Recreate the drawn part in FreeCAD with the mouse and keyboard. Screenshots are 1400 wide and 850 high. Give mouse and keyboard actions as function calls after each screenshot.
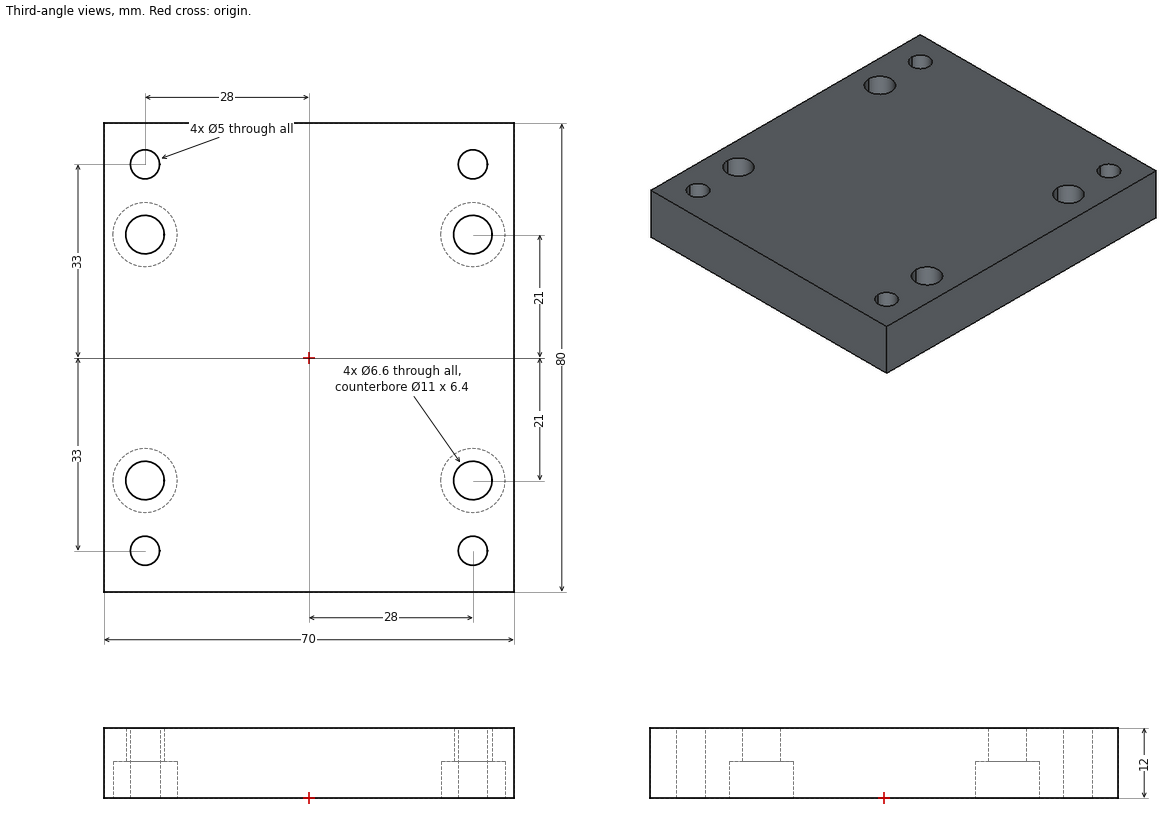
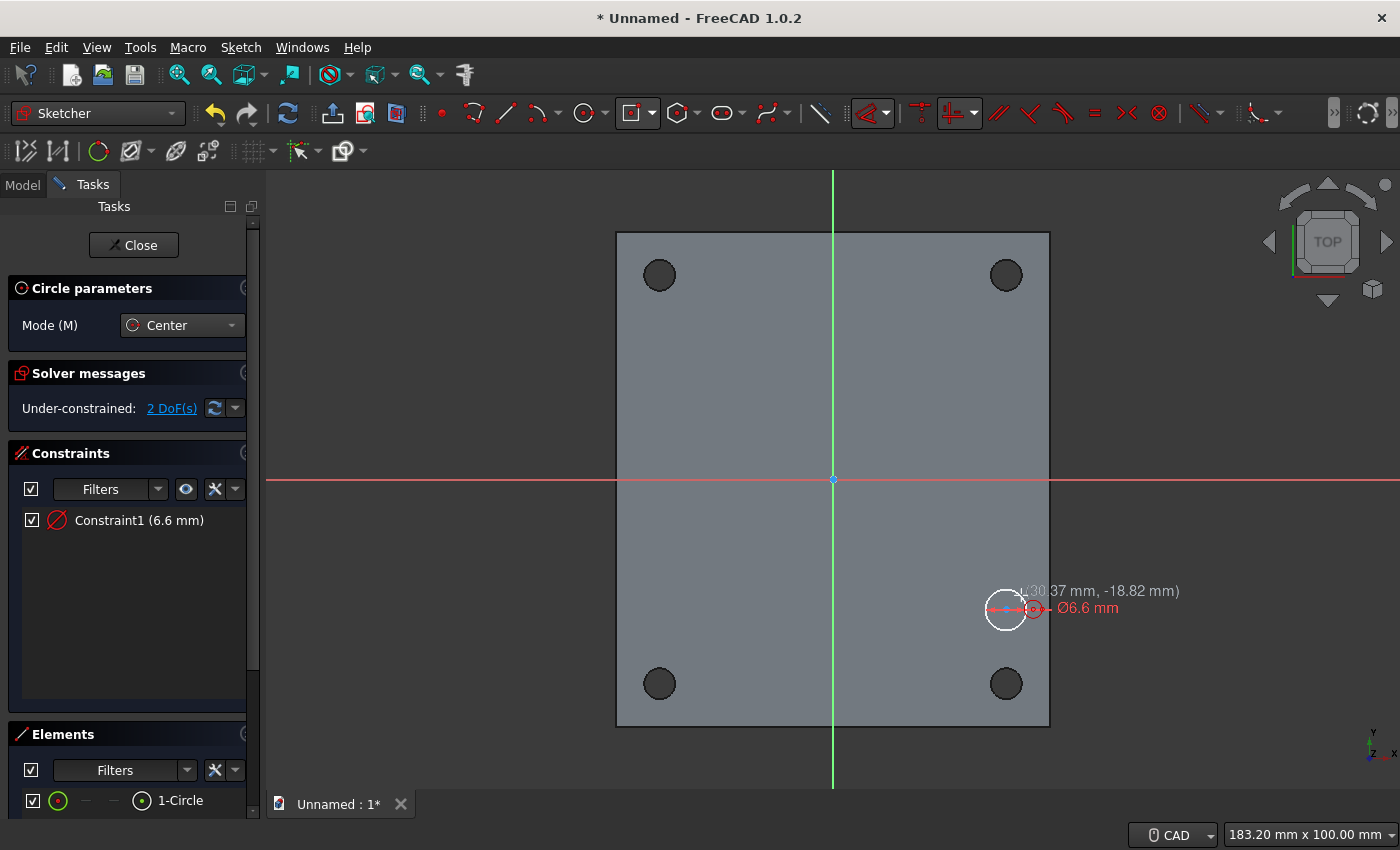
click(1006, 350)
move(1021, 335)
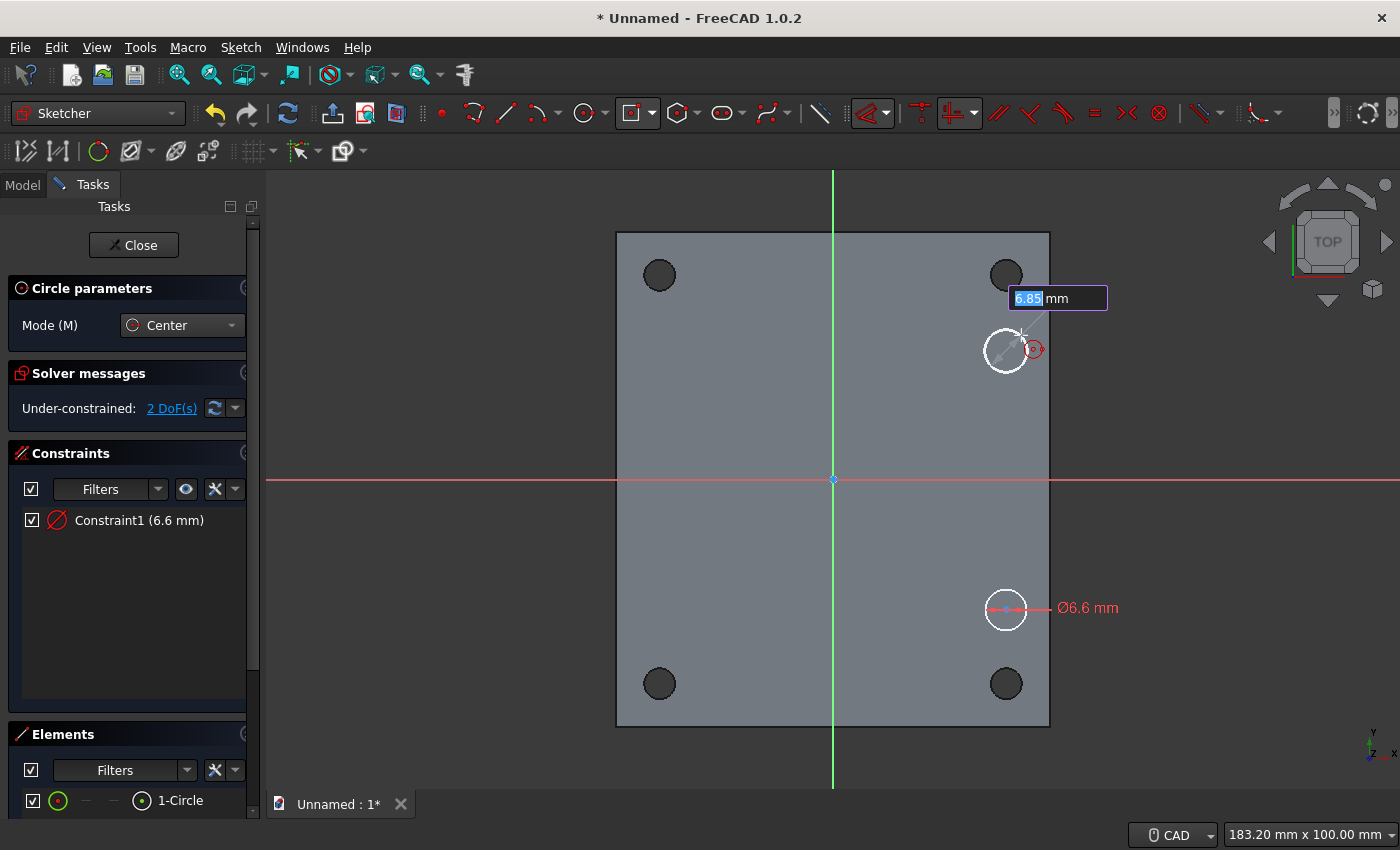
text(6.6)
key(Return)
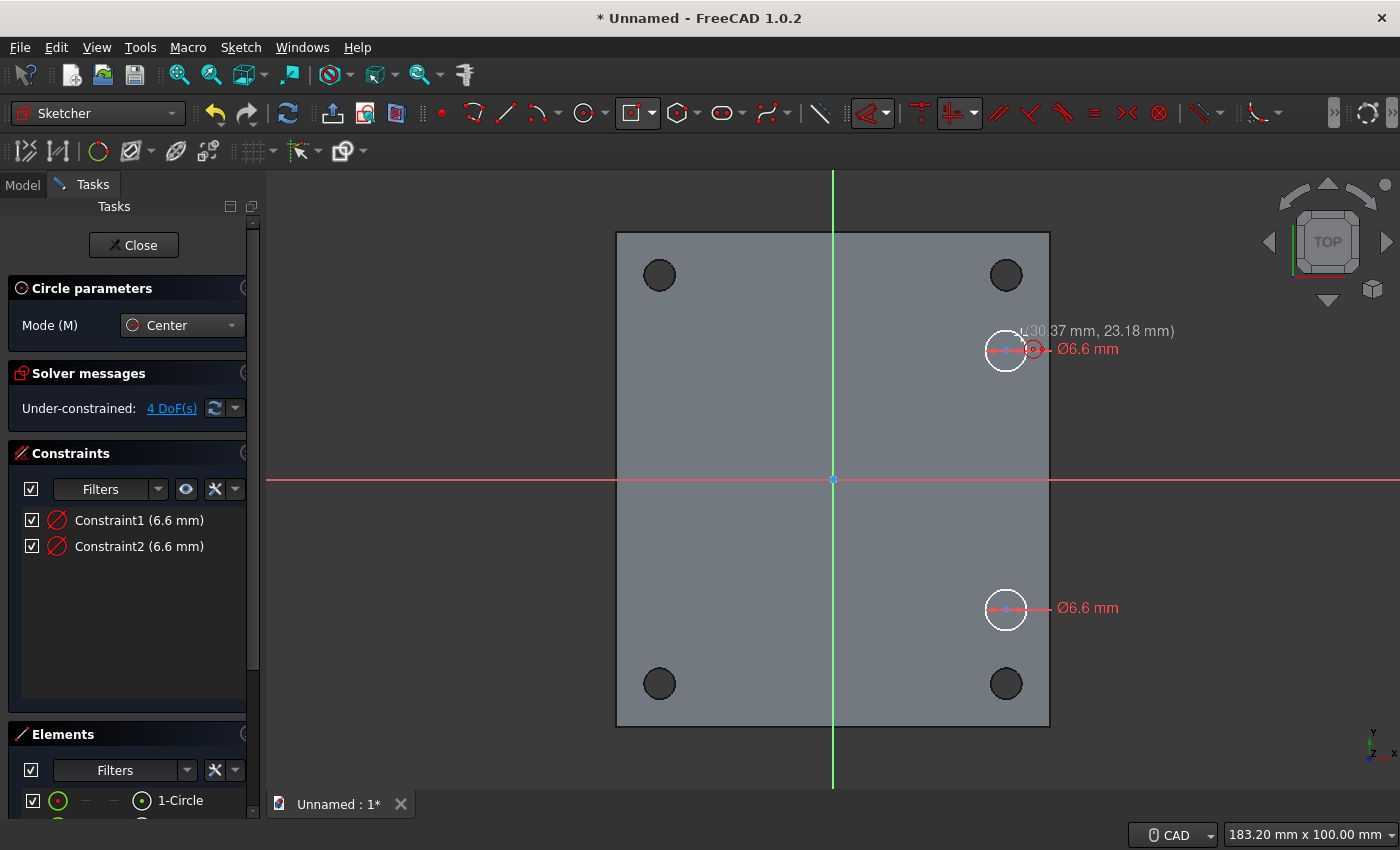
click(660, 609)
move(674, 595)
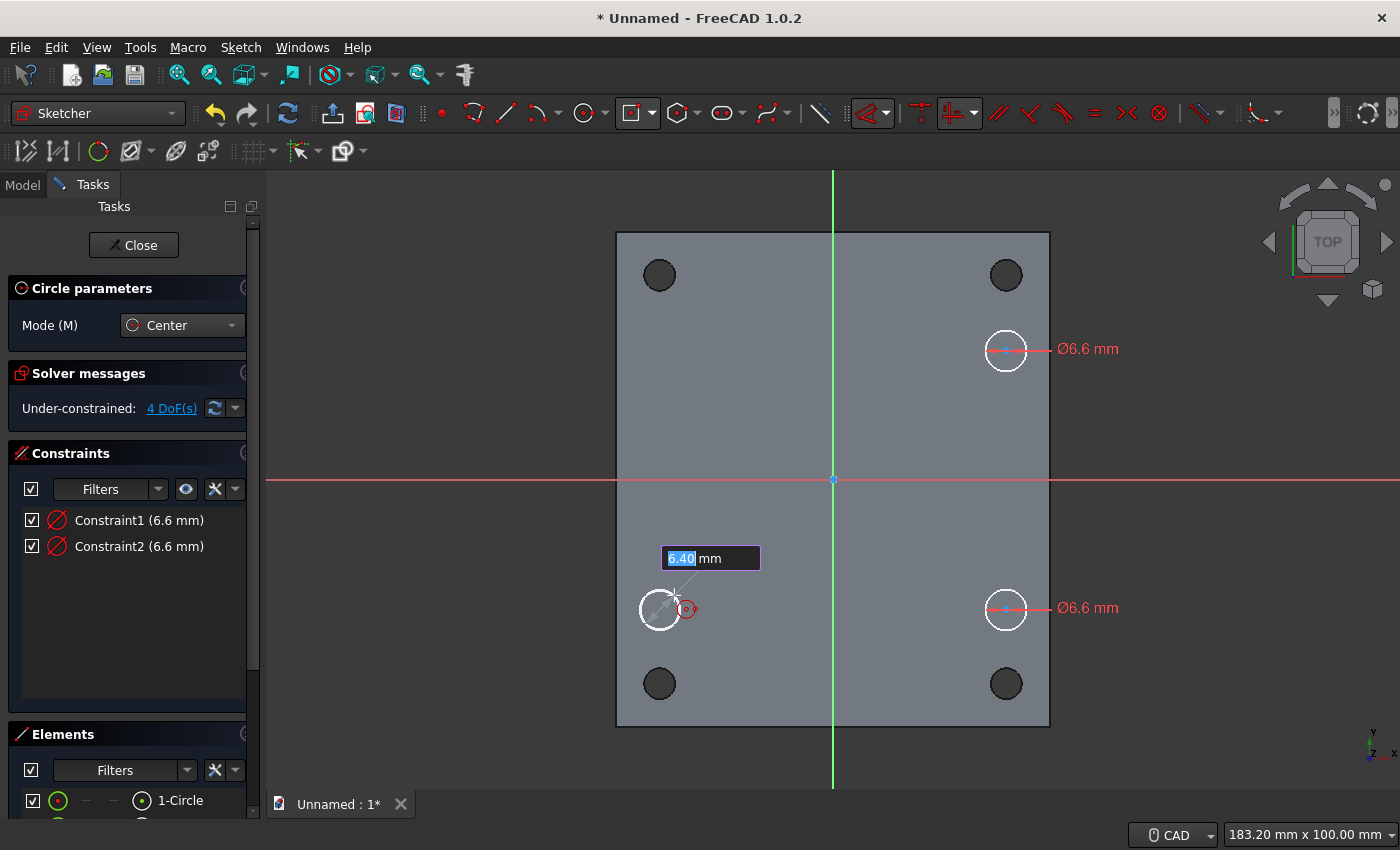
text(6.6)
key(Return)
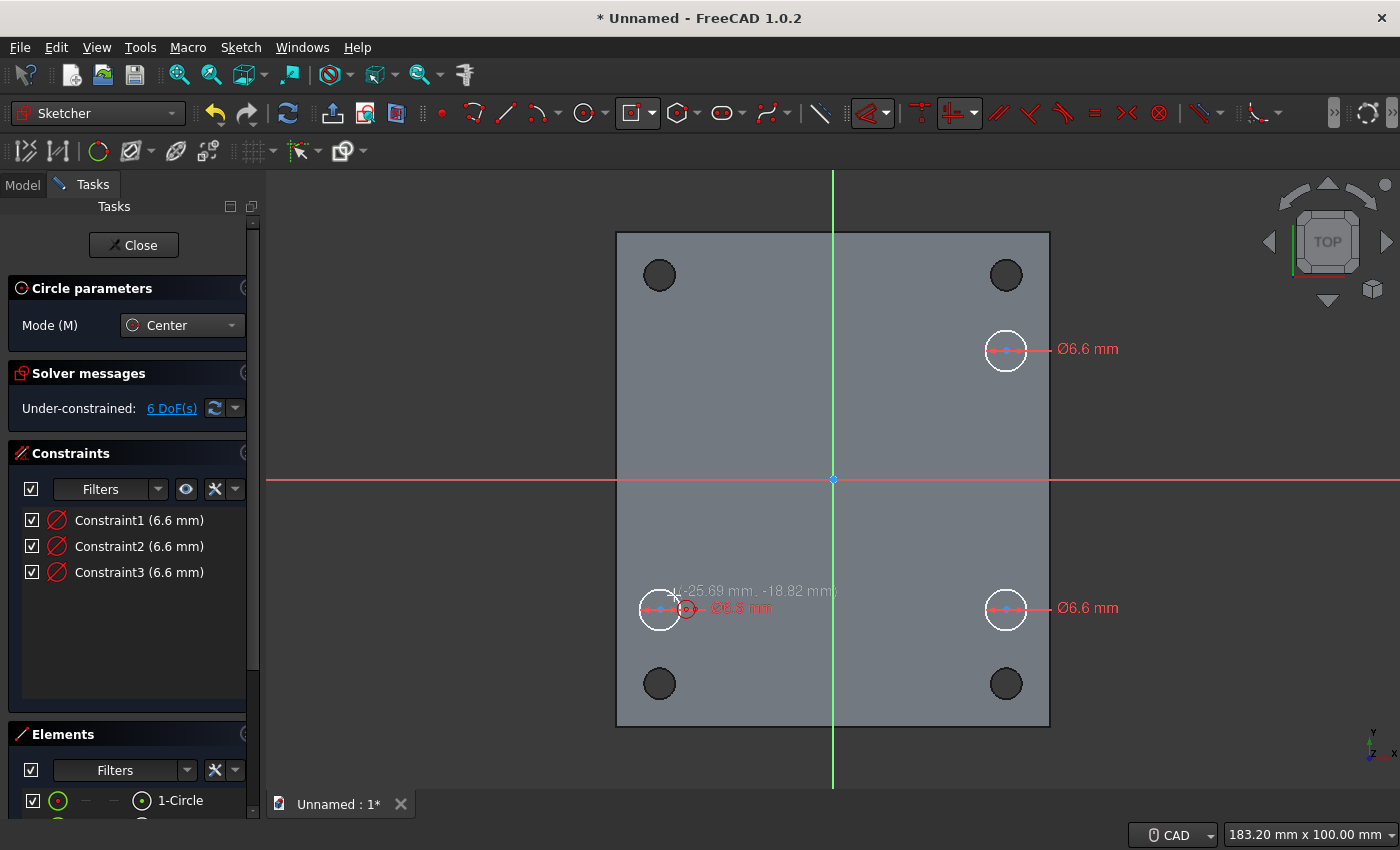
click(660, 350)
move(674, 335)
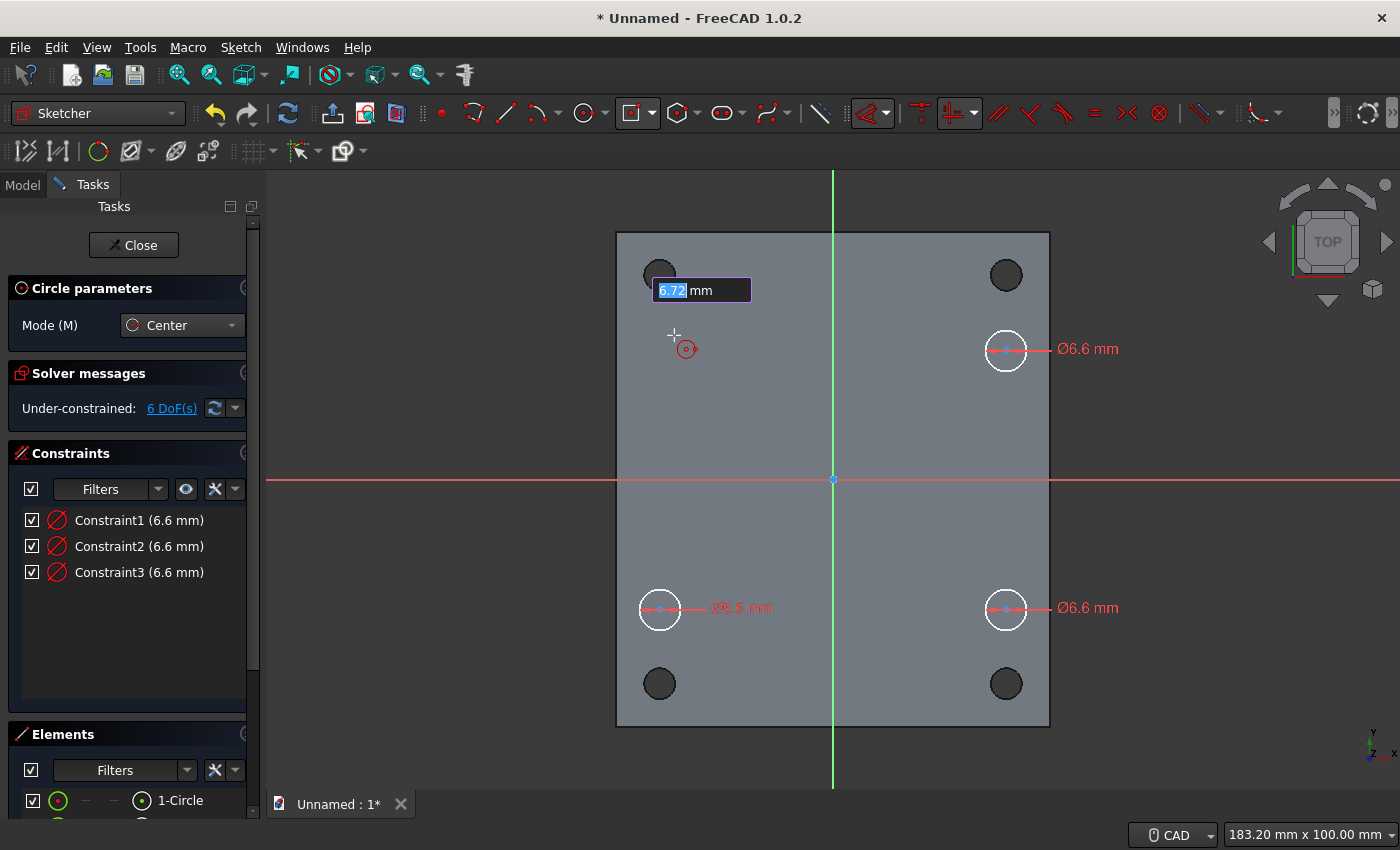
text(6.6)
key(Return)
key(Escape)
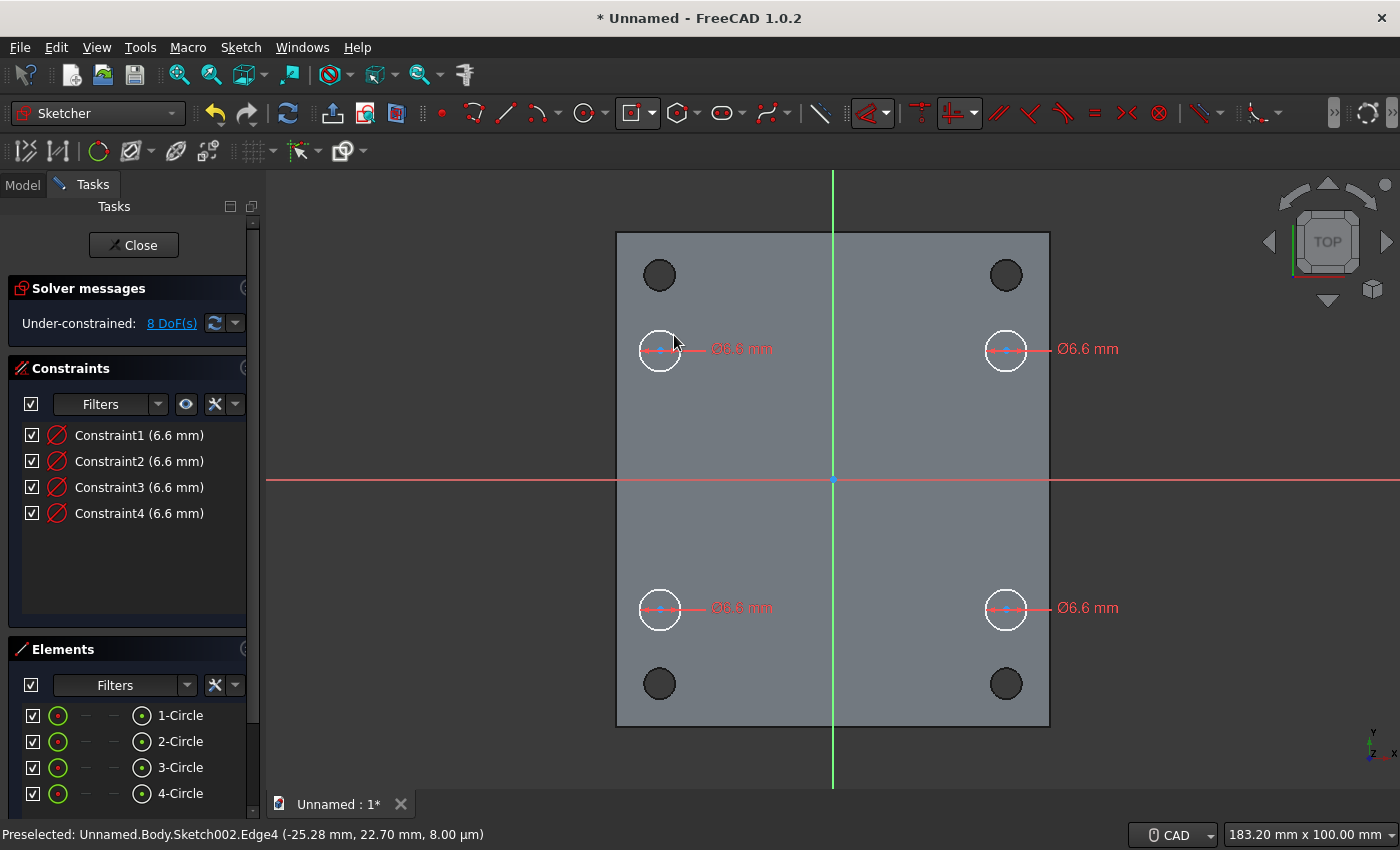
click(1006, 610)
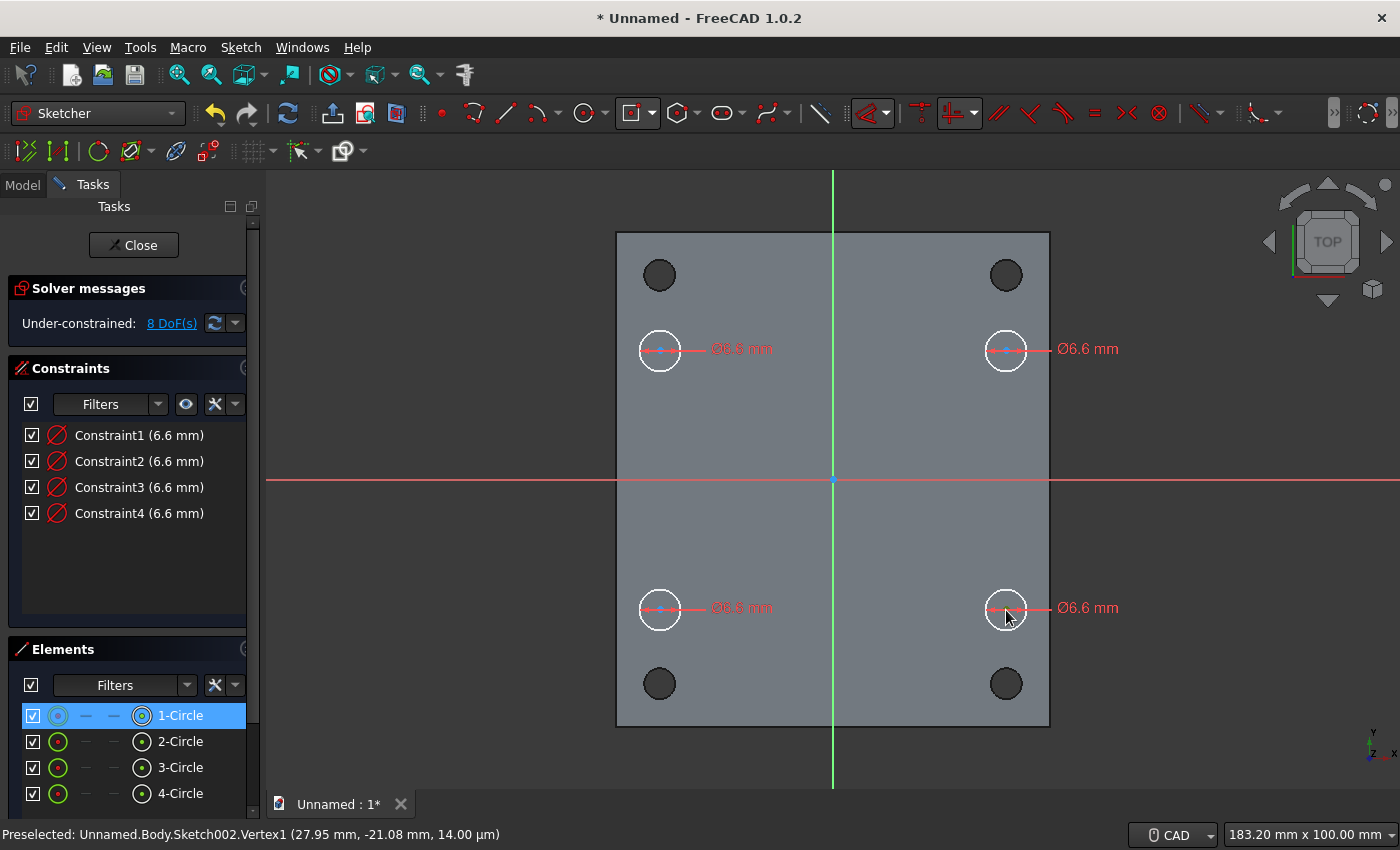
click(1006, 351)